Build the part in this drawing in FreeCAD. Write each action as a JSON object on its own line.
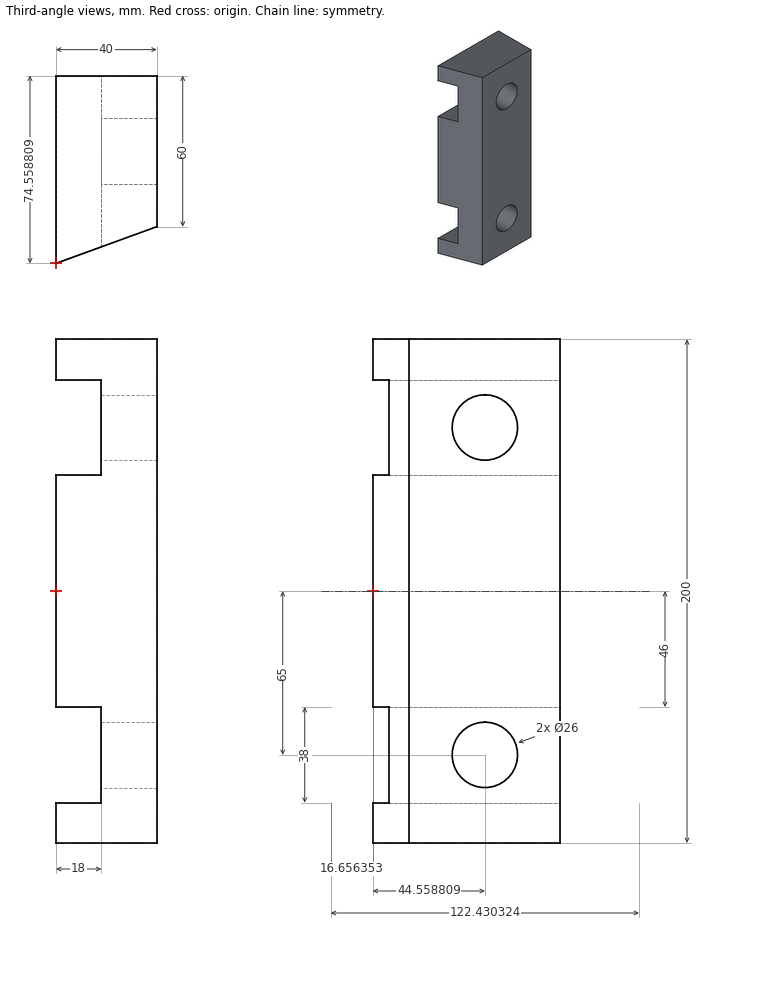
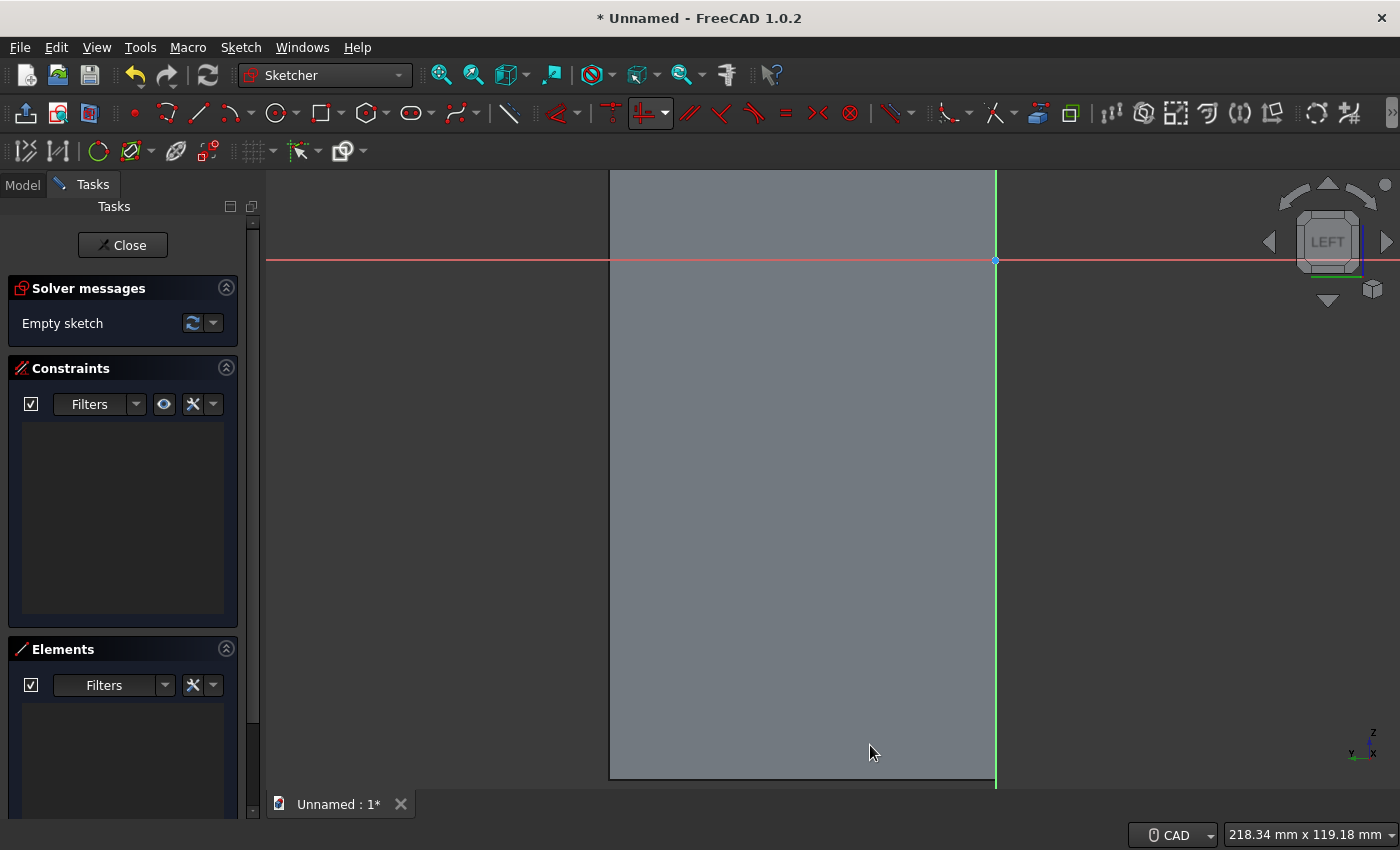
{"action": "left_click", "coordinate": [322, 114]}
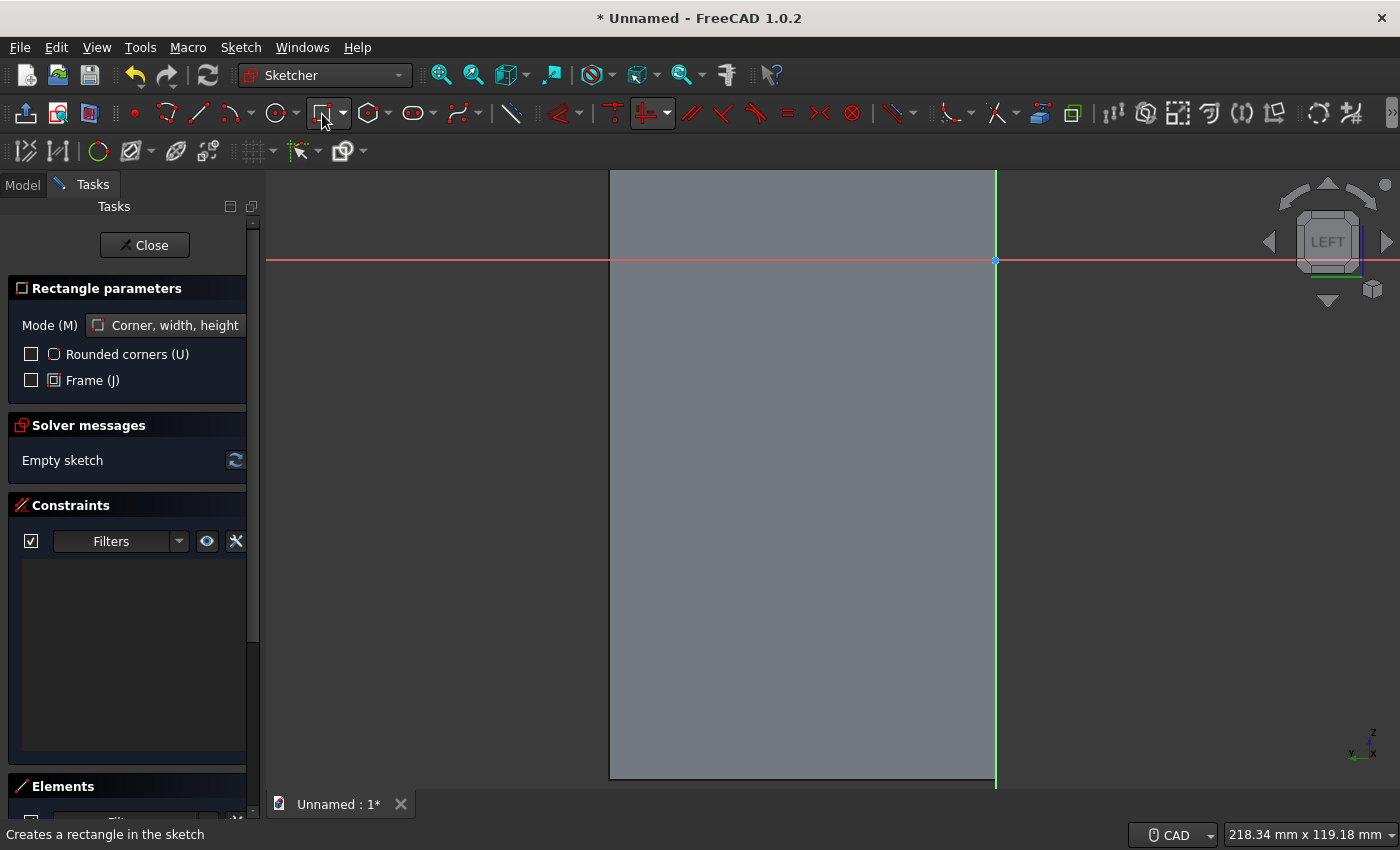
{"action": "left_click", "coordinate": [446, 499]}
{"action": "mouse_move", "coordinate": [1082, 697]}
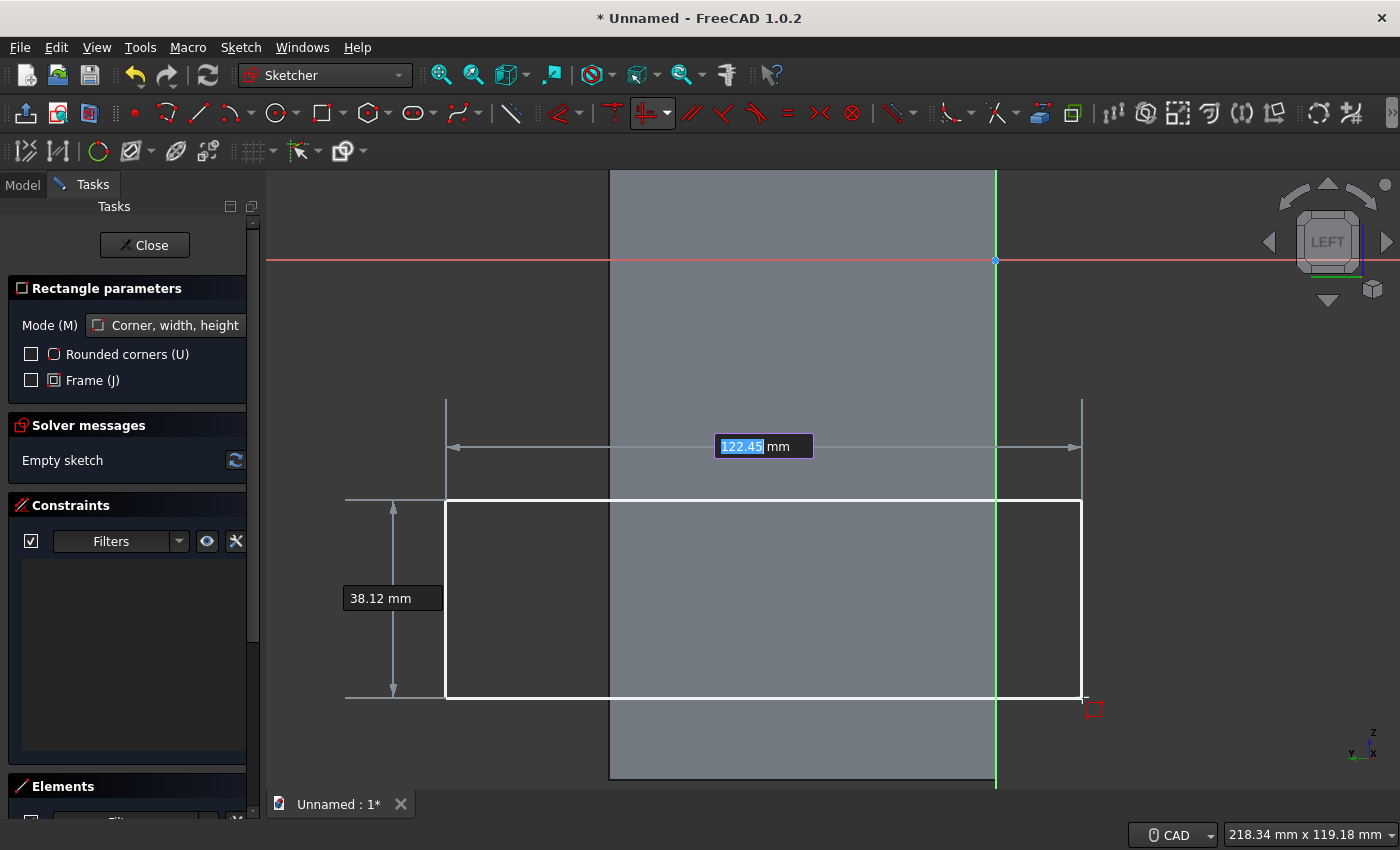
{"action": "type", "text": "122.430324"}
{"action": "key", "text": "Tab"}
{"action": "type", "text": "38"}
{"action": "key", "text": "Return"}
{"action": "key", "text": "Escape"}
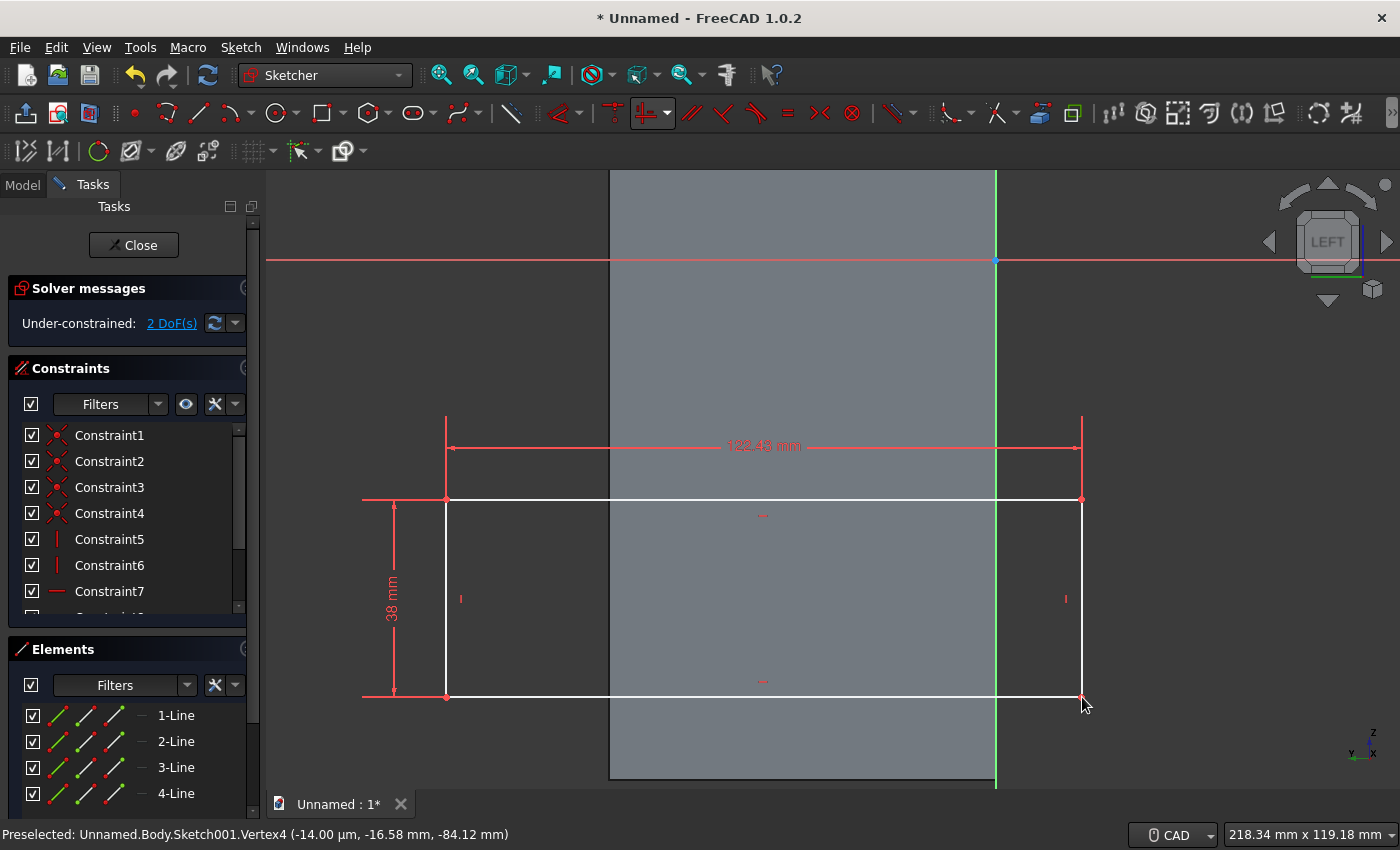
{"action": "left_click", "coordinate": [558, 114]}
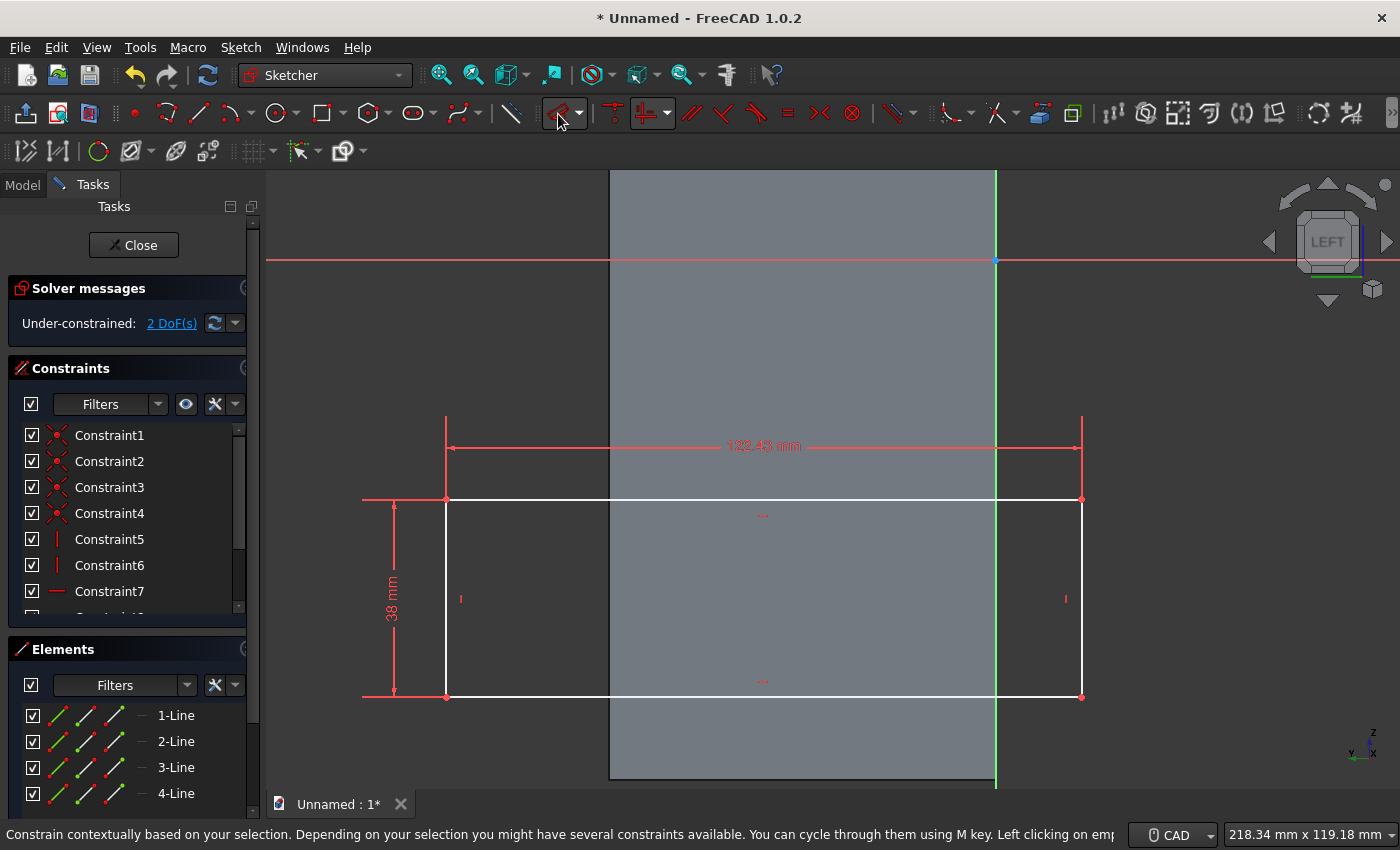
{"action": "left_click", "coordinate": [446, 500]}
{"action": "left_click", "coordinate": [412, 380]}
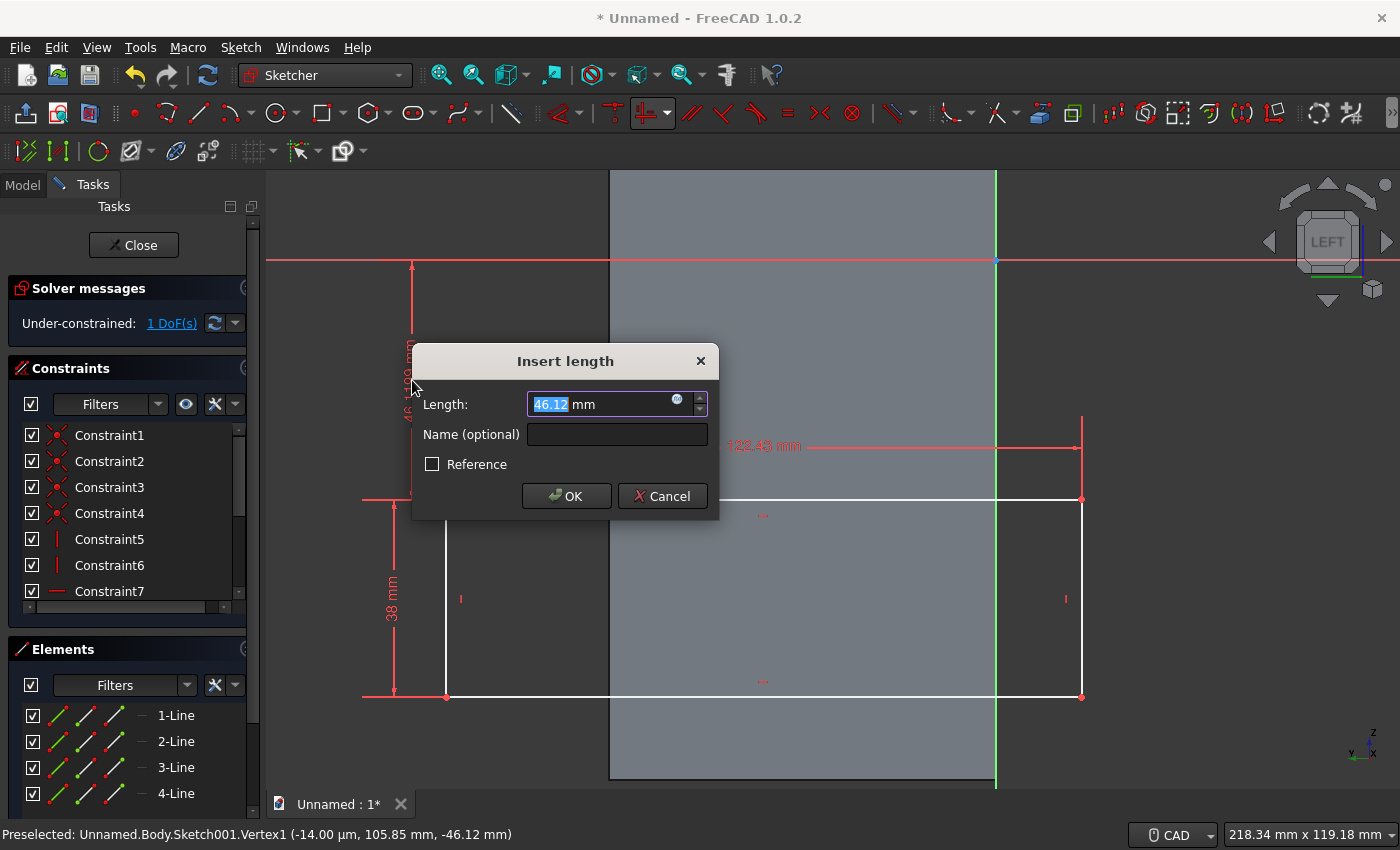
{"action": "type", "text": "46"}
{"action": "key", "text": "Return"}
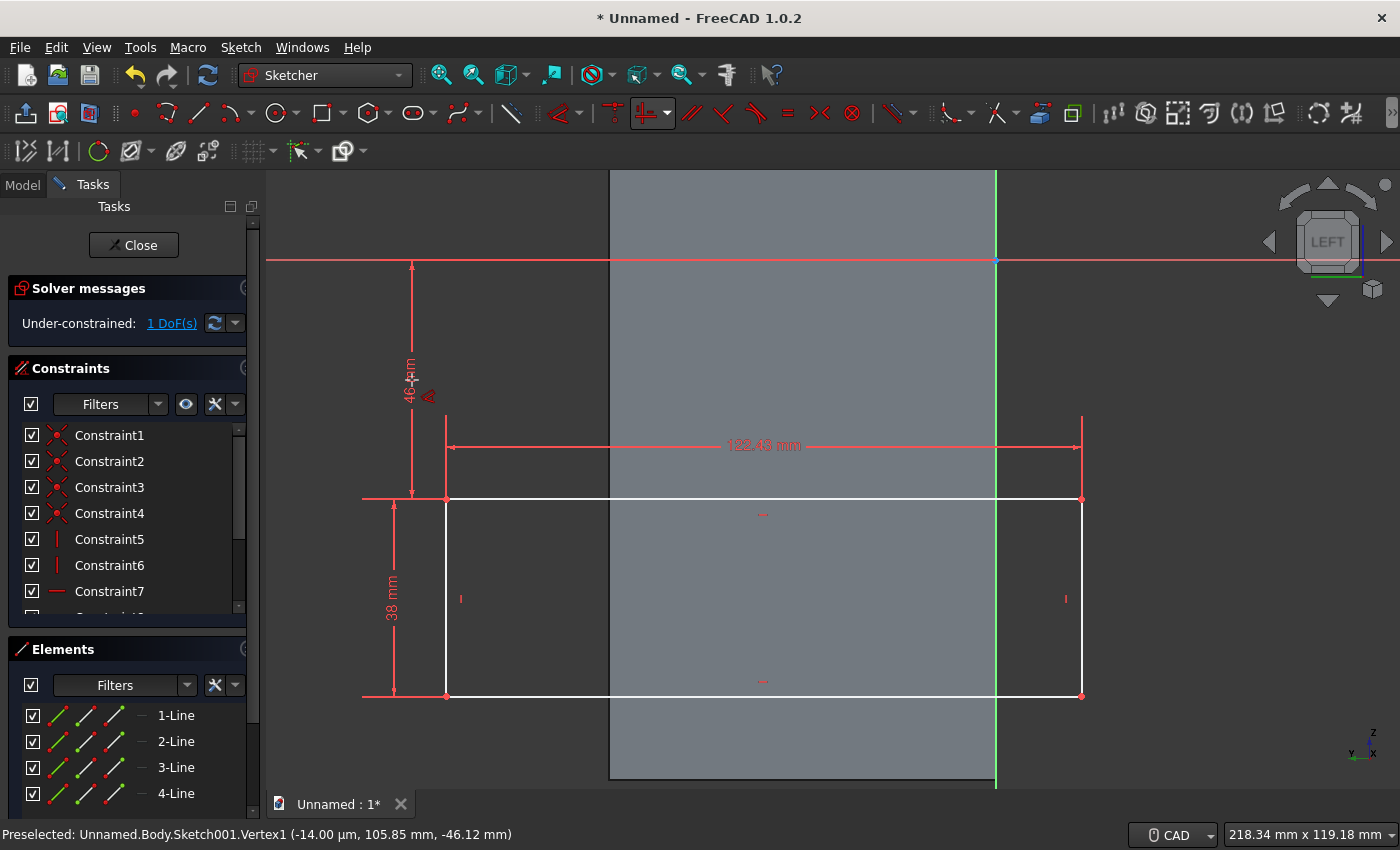
{"action": "left_click", "coordinate": [1082, 697]}
{"action": "left_click", "coordinate": [1039, 226]}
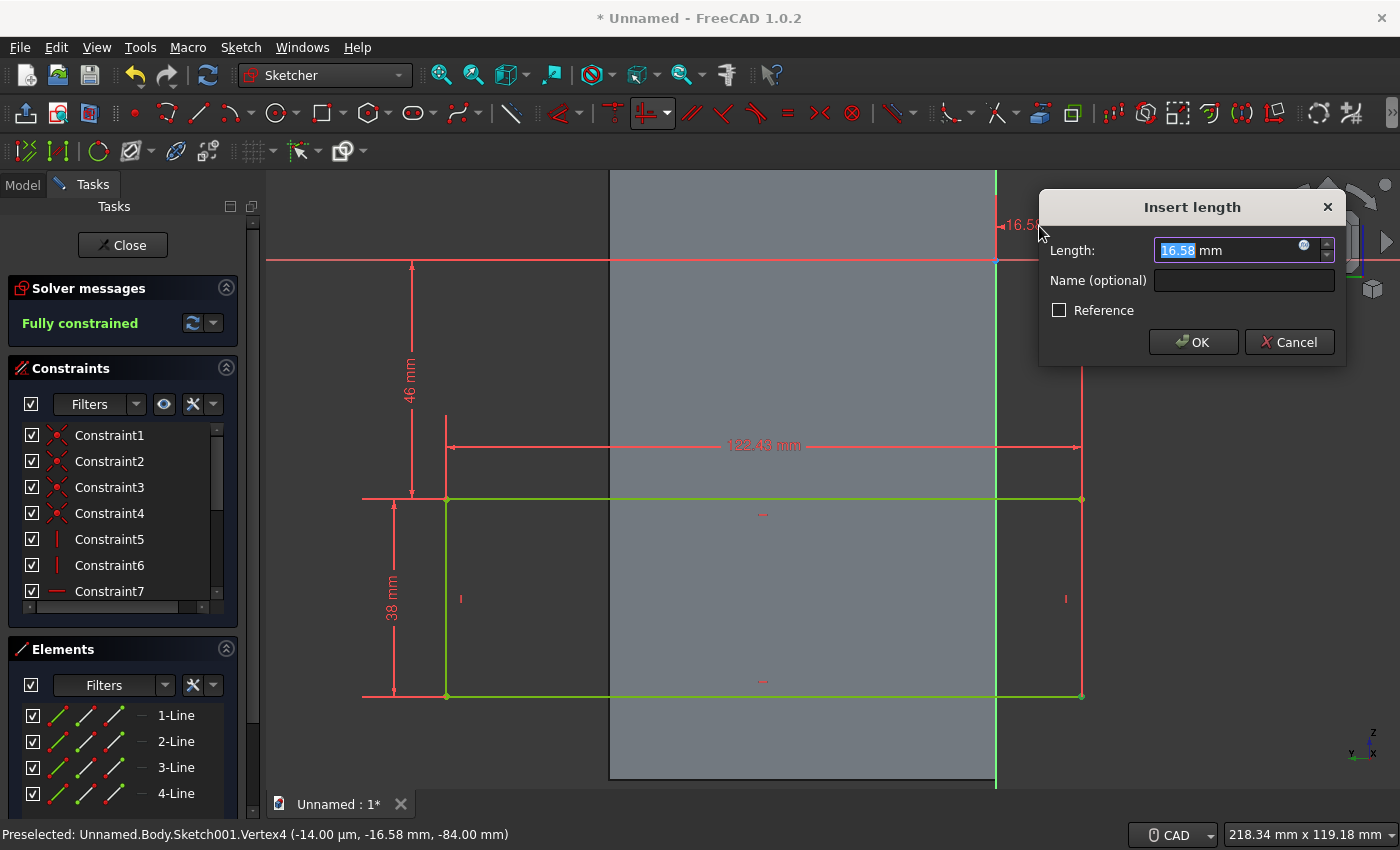
{"action": "type", "text": "16.656353"}
{"action": "key", "text": "Return"}
{"action": "key", "text": "Escape"}